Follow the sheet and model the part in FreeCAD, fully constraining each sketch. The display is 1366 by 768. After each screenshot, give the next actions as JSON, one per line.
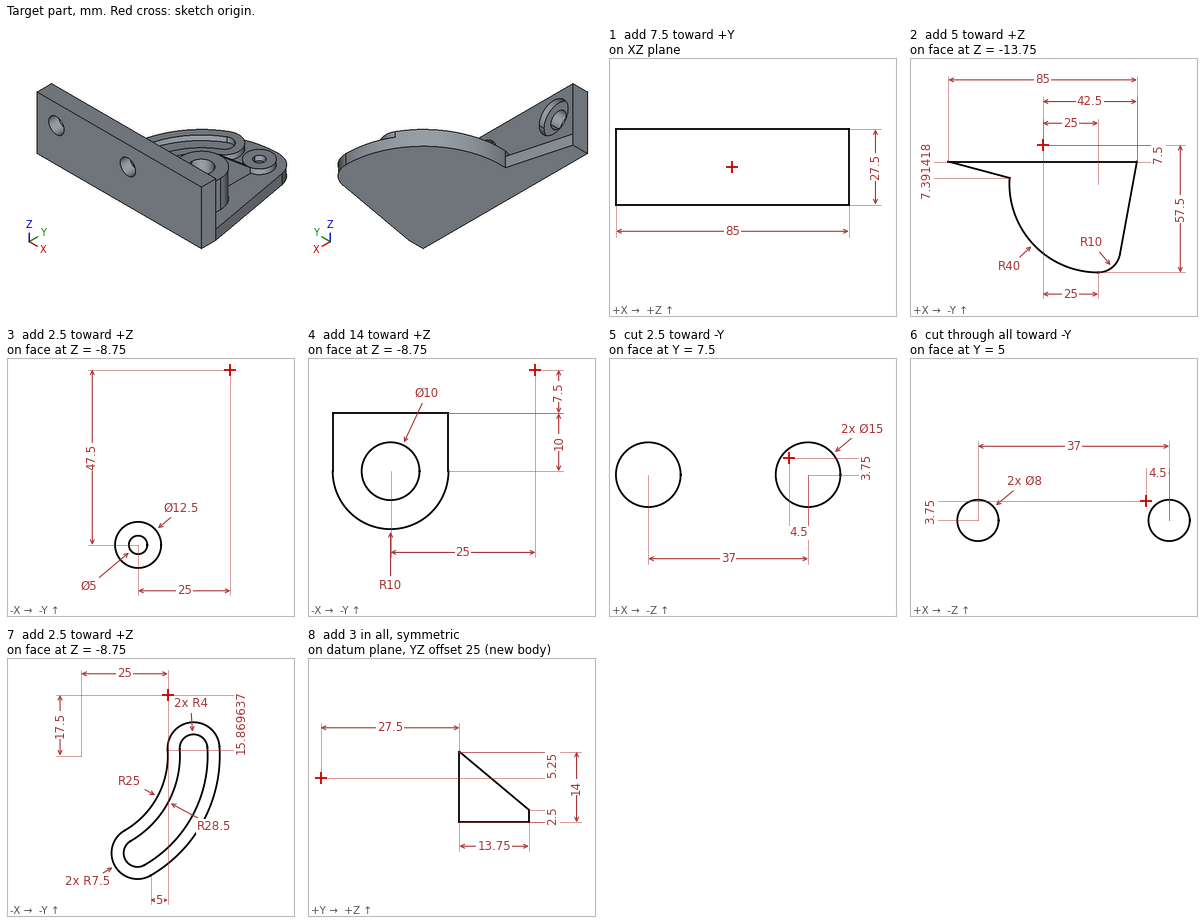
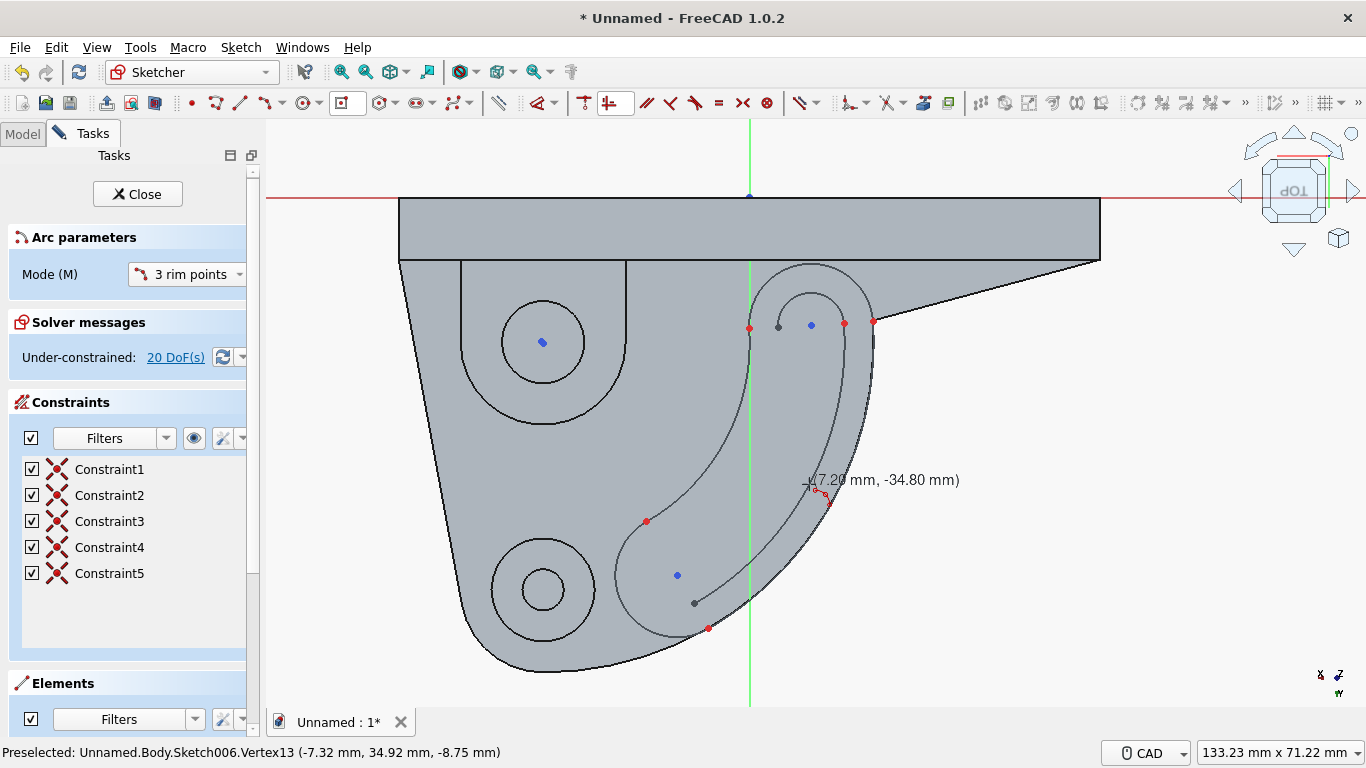
{"action": "left_click", "coordinate": [694, 604]}
{"action": "left_click", "coordinate": [661, 546]}
{"action": "left_click", "coordinate": [649, 591]}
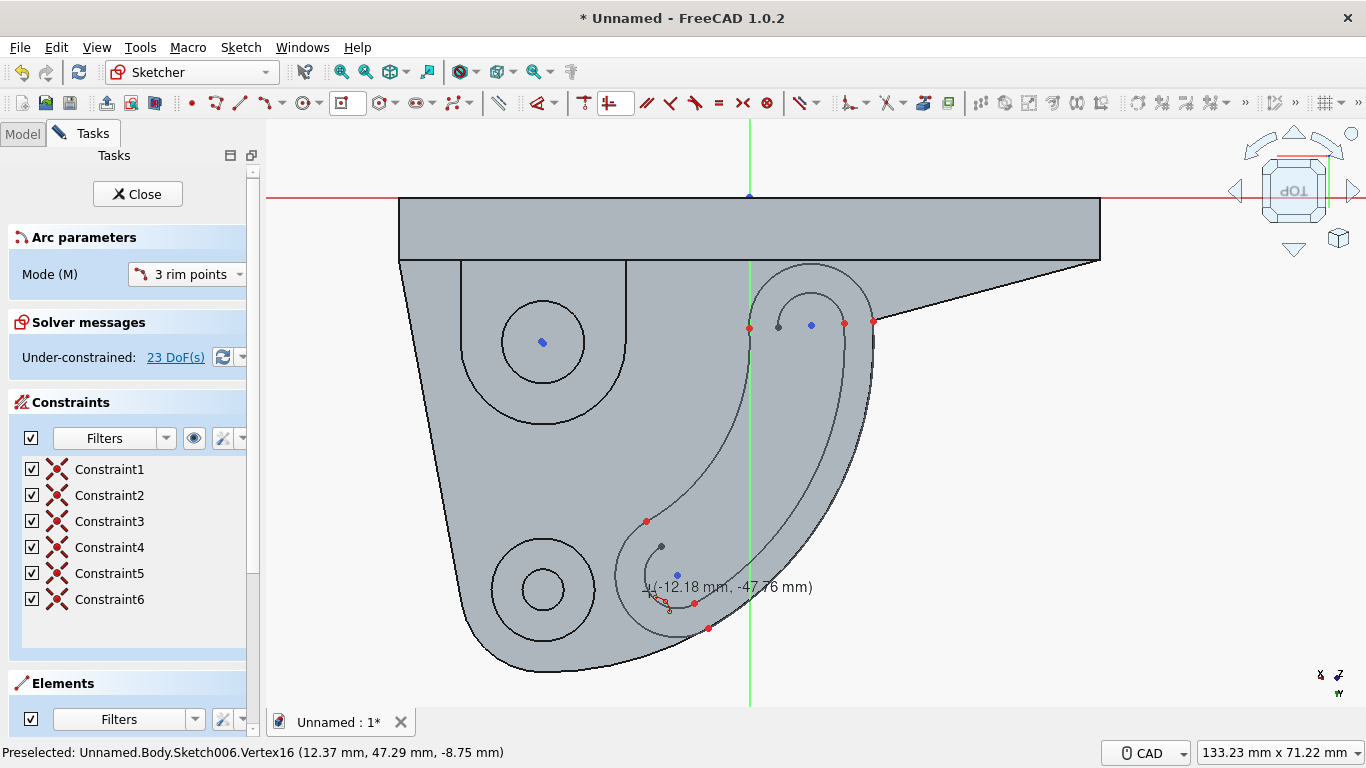
{"action": "left_click", "coordinate": [661, 547]}
{"action": "left_click", "coordinate": [778, 328]}
{"action": "left_click", "coordinate": [721, 496]}
{"action": "key", "text": "Escape"}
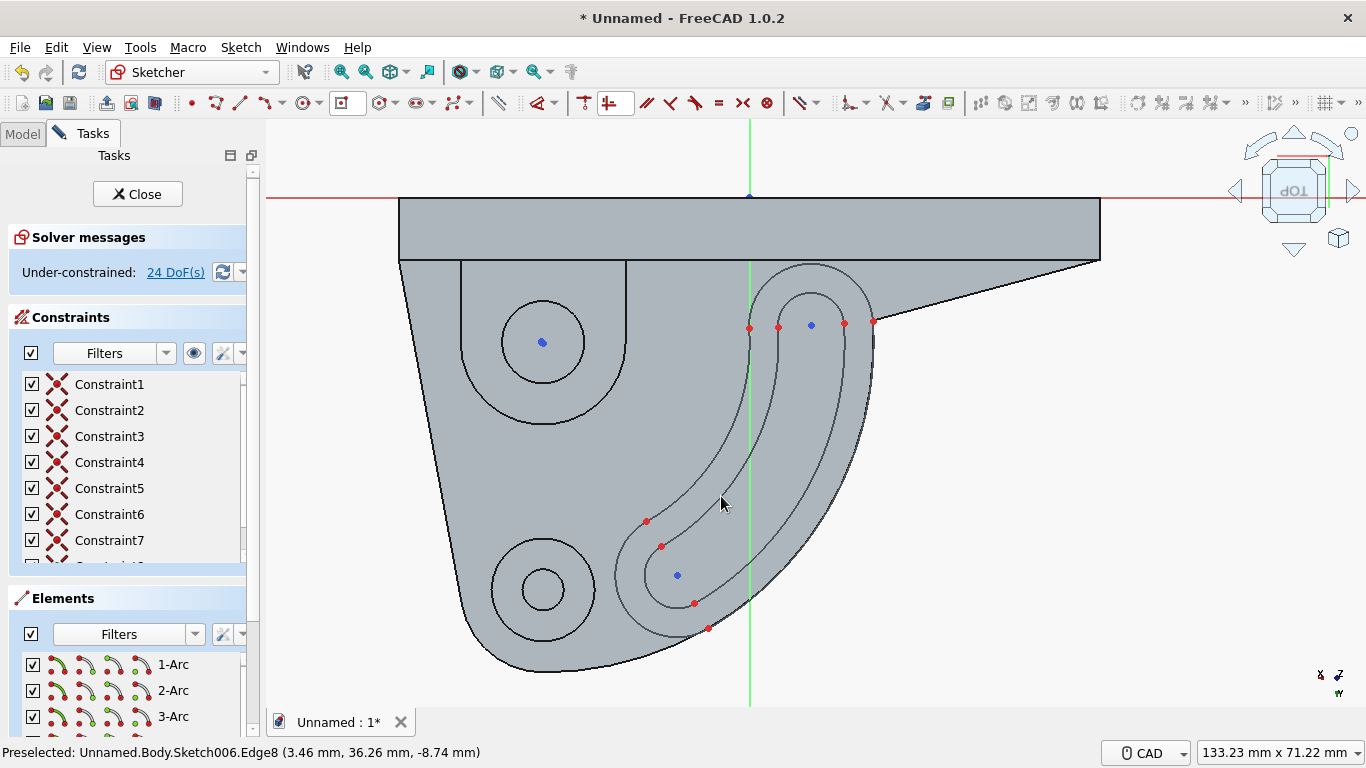
{"action": "left_click", "coordinate": [699, 478]}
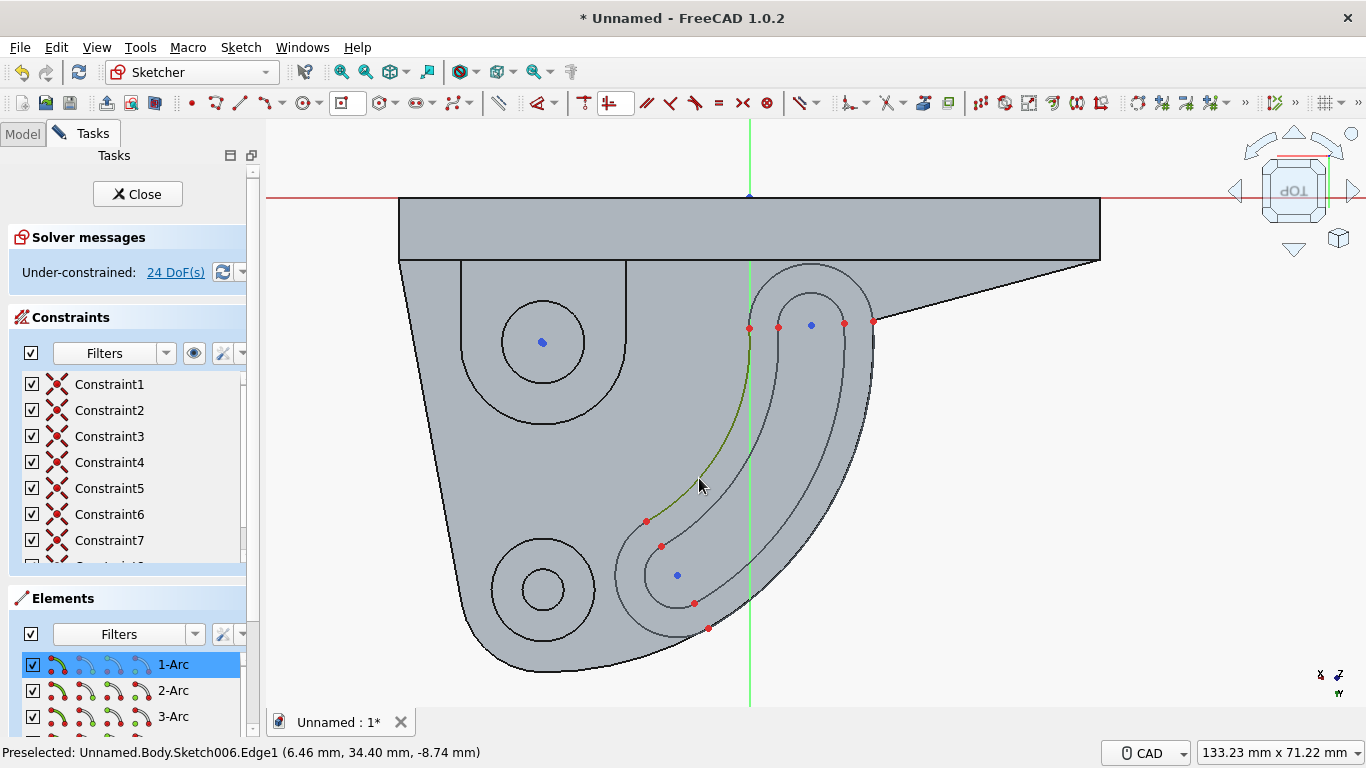
{"action": "left_click", "coordinate": [616, 569]}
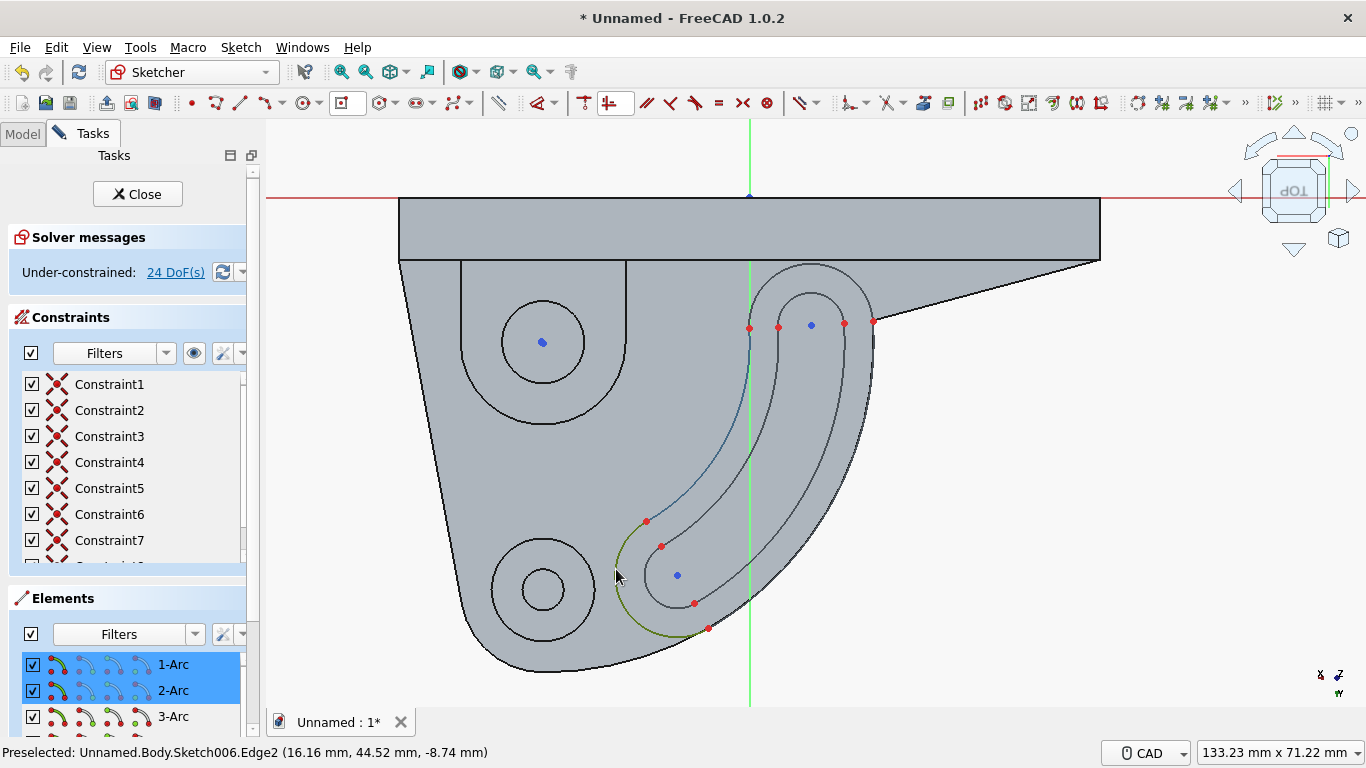
{"action": "left_click", "coordinate": [696, 104]}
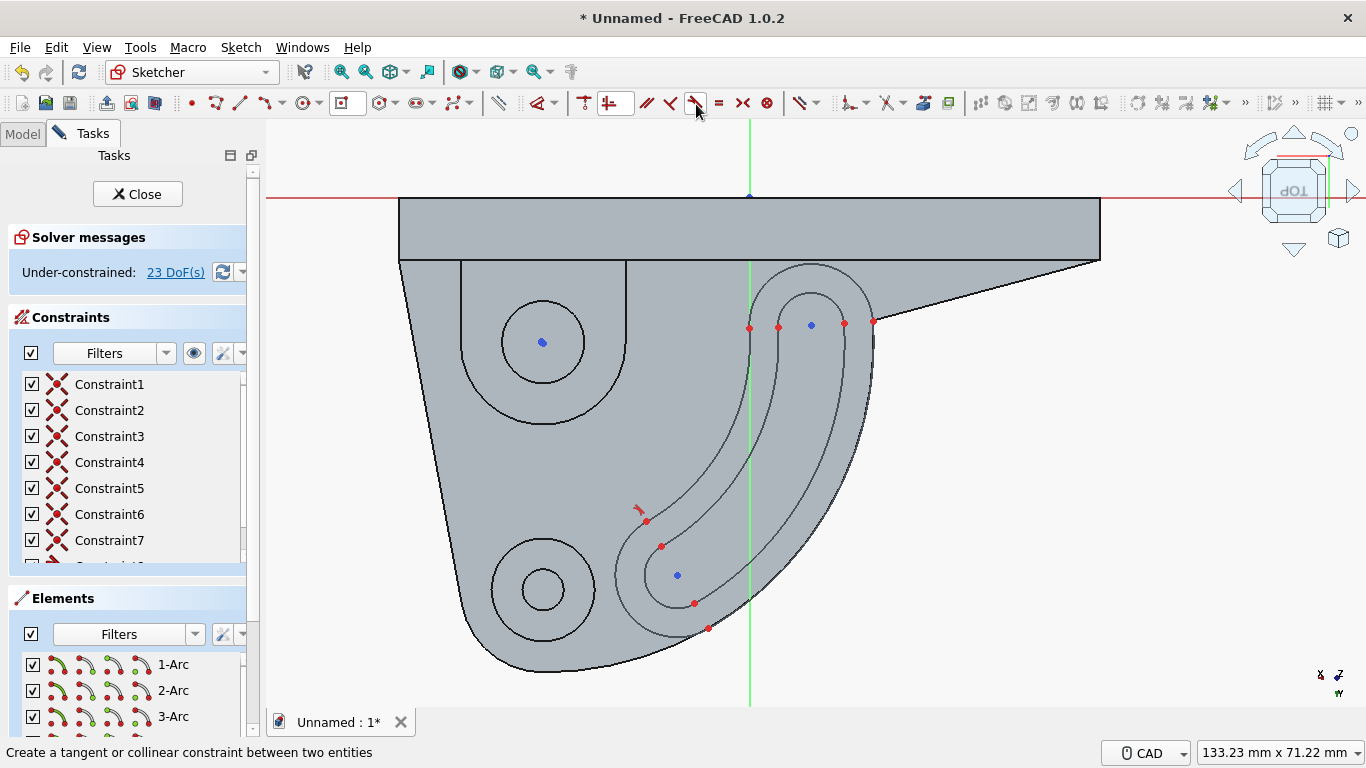
{"action": "left_click", "coordinate": [700, 478]}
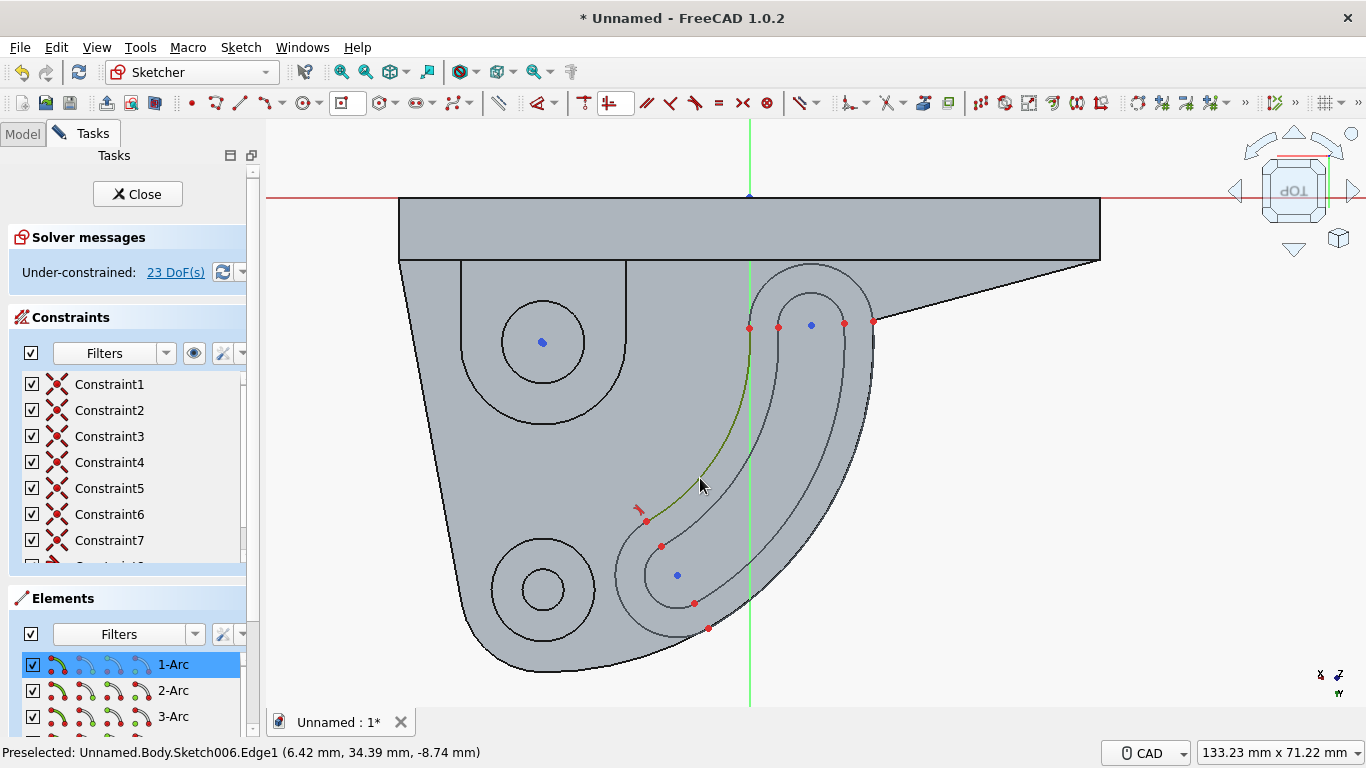
{"action": "left_click", "coordinate": [845, 274]}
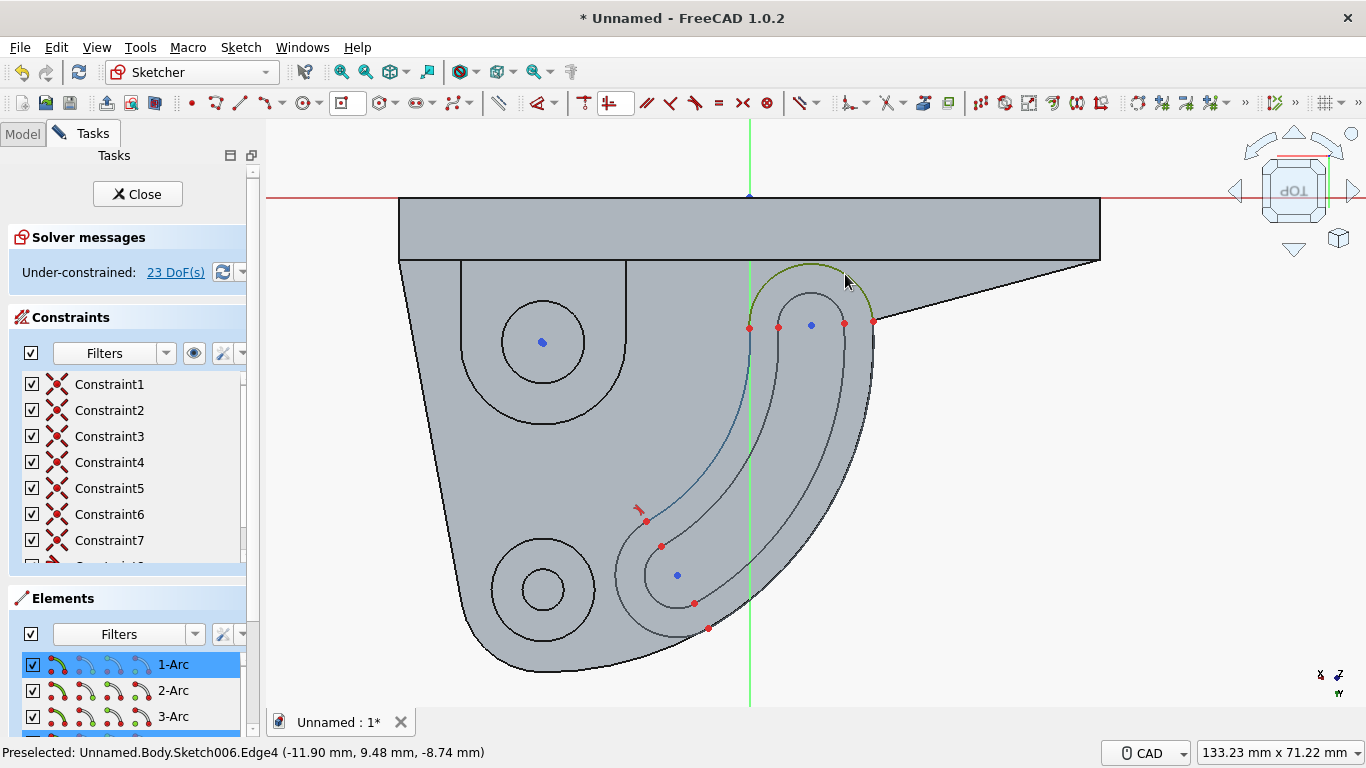
{"action": "left_click", "coordinate": [696, 104]}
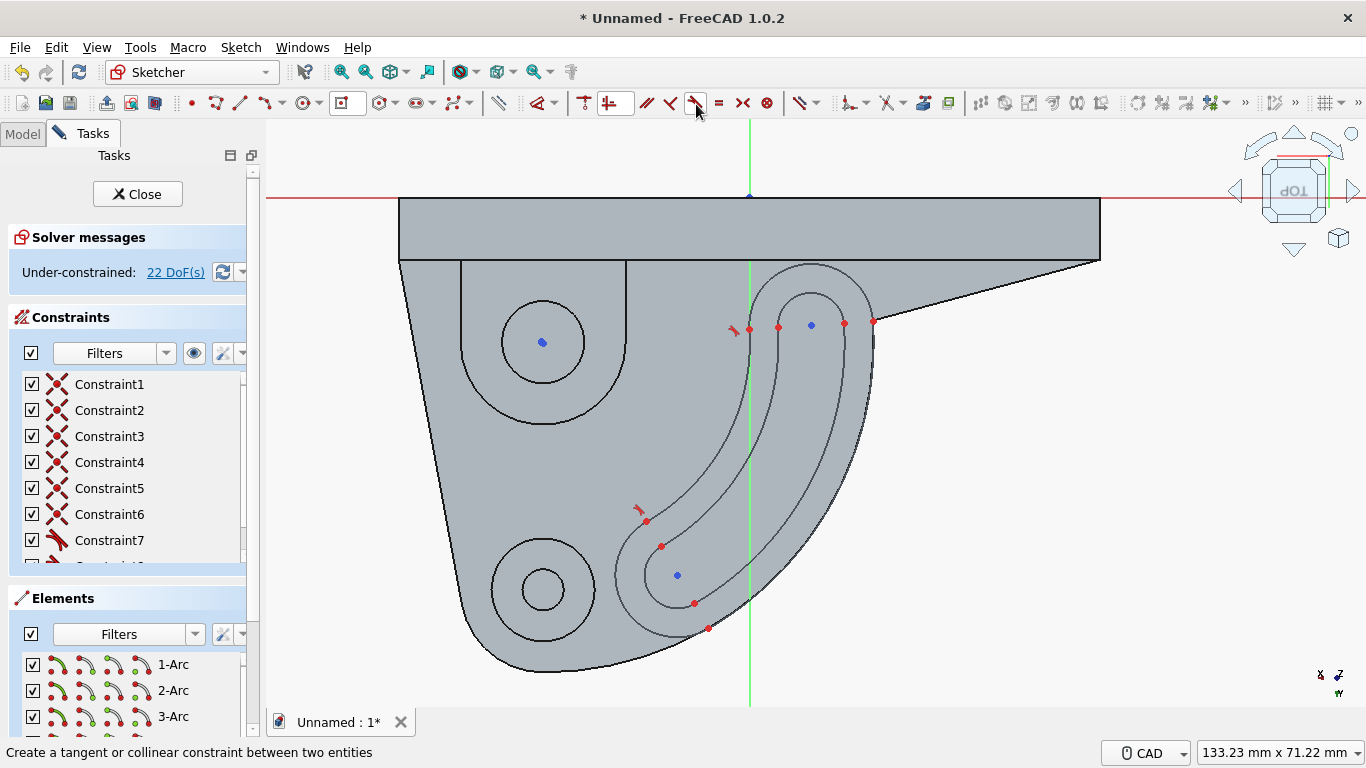
{"action": "left_click", "coordinate": [616, 569]}